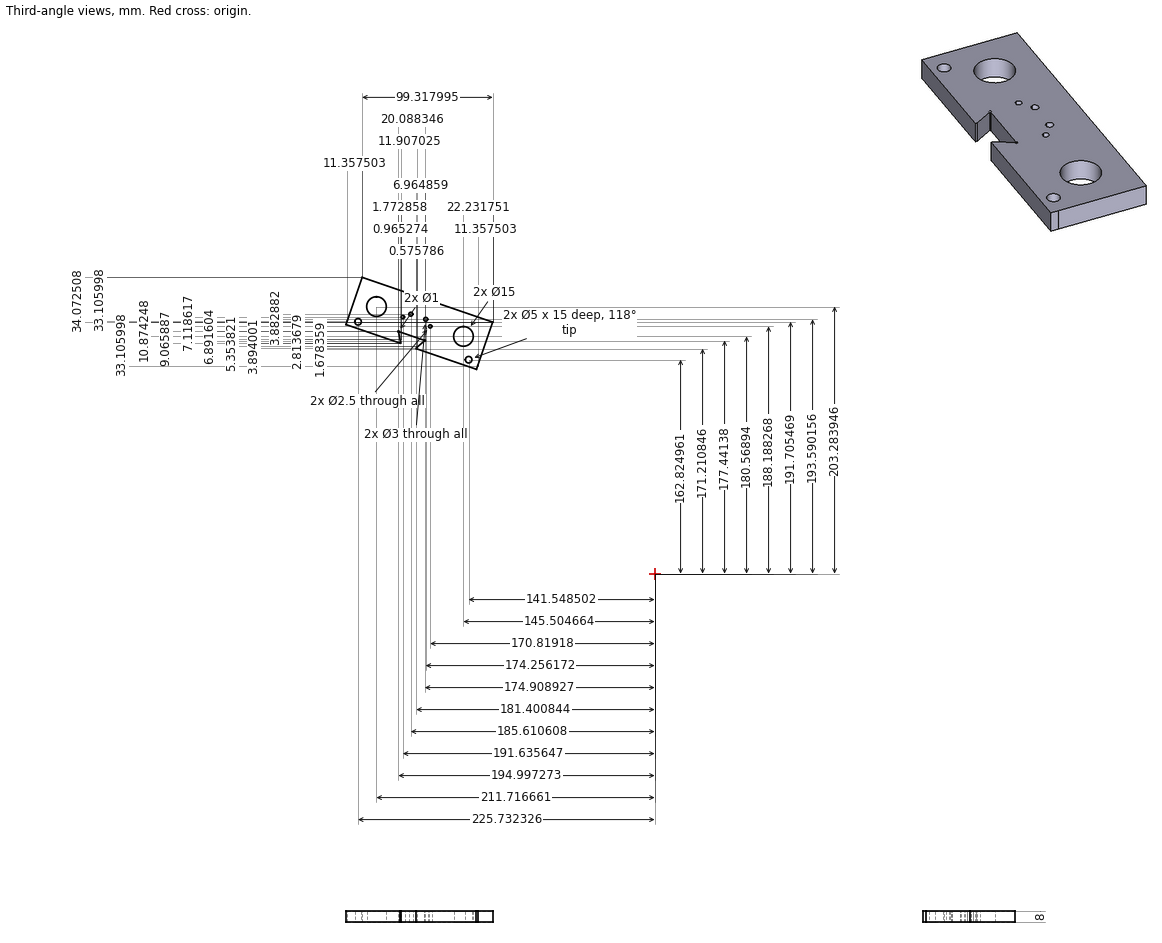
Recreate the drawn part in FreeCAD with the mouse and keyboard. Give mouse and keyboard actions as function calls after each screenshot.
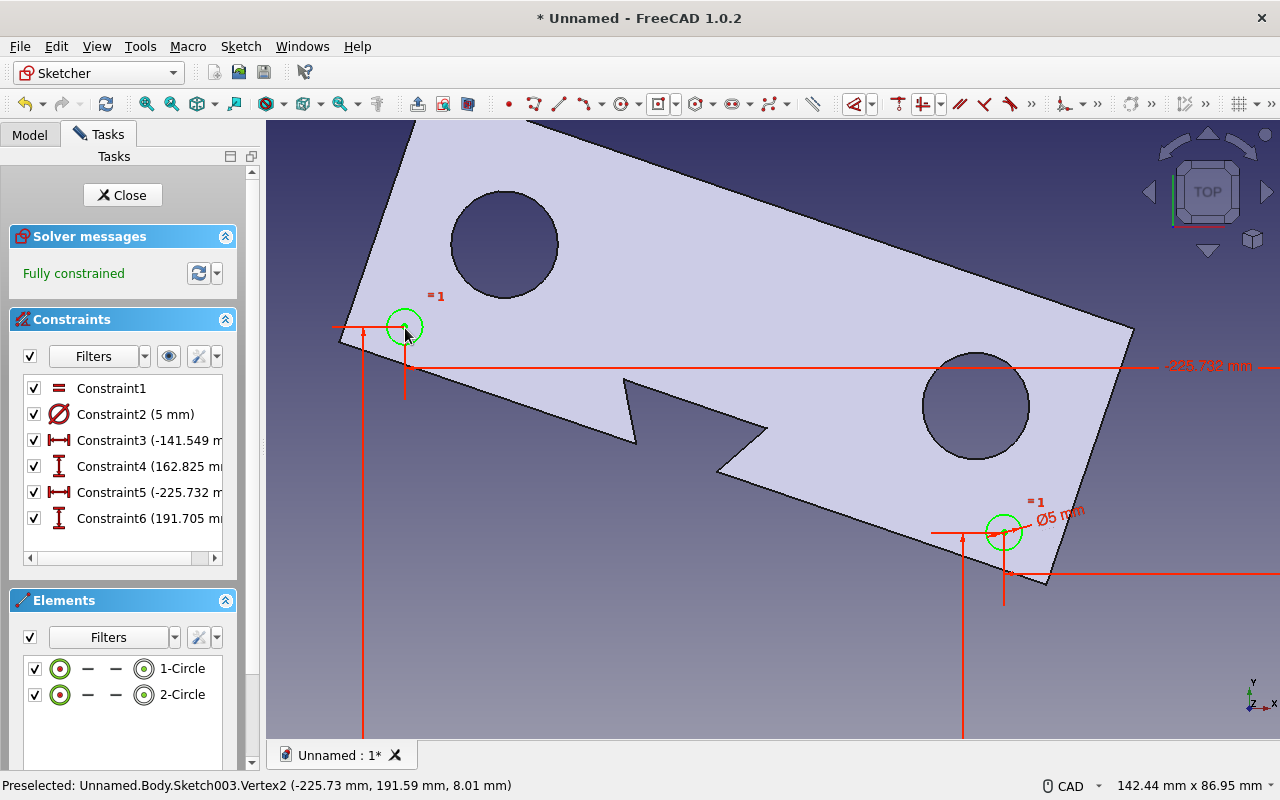
click(123, 195)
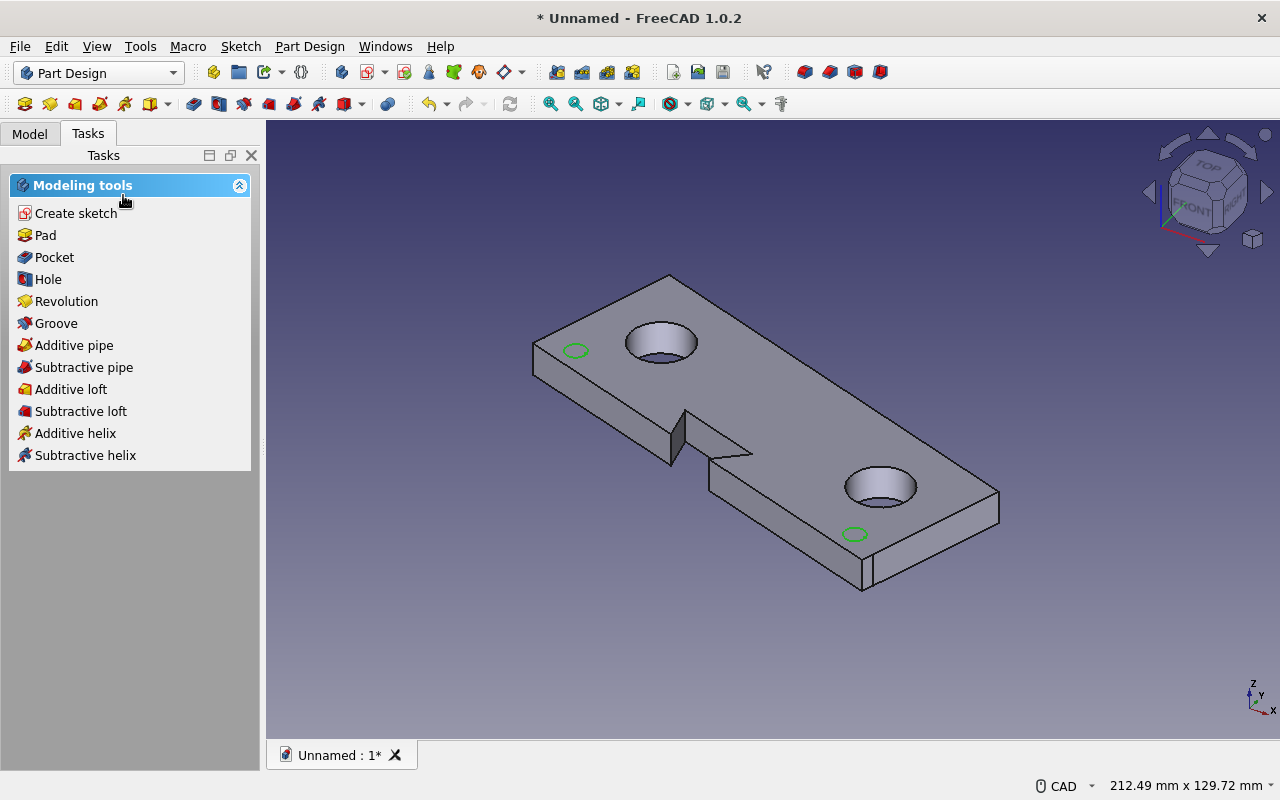
click(219, 104)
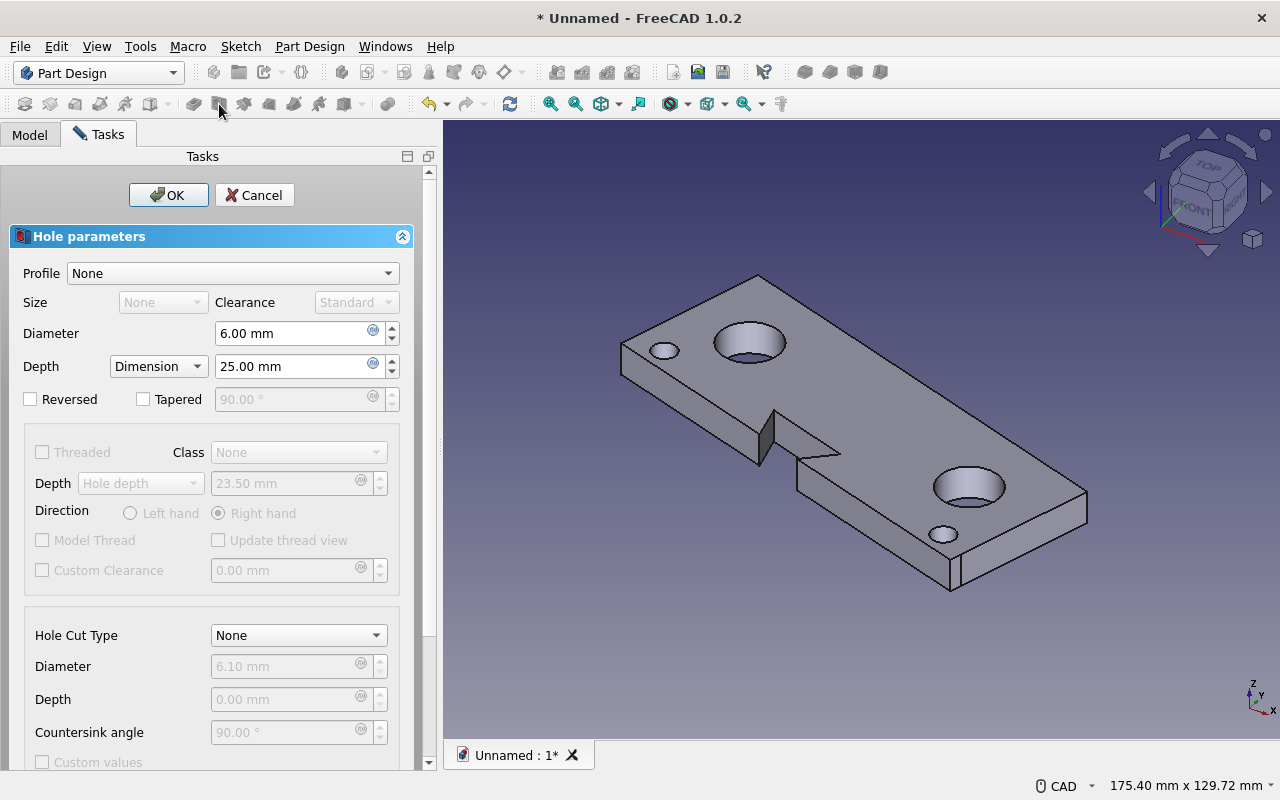
triple_click(300, 334)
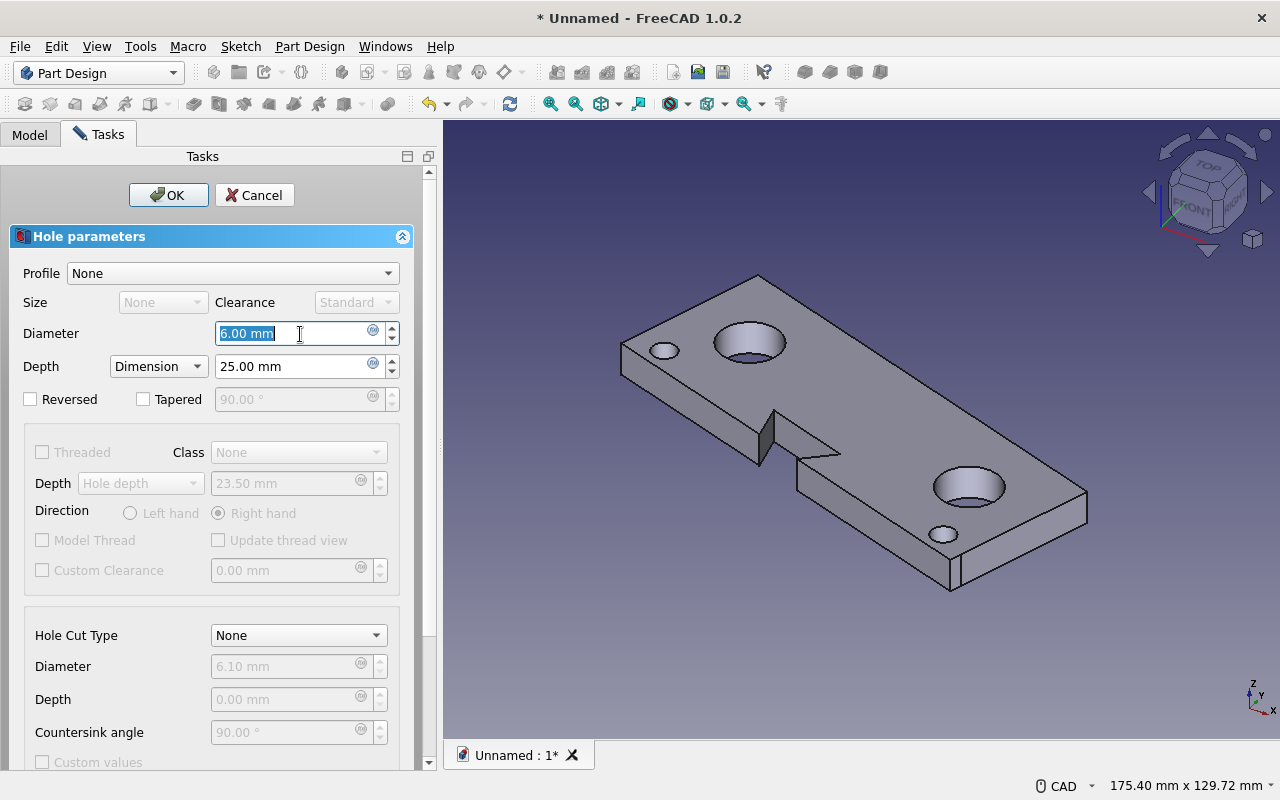
text(5)
key(Tab)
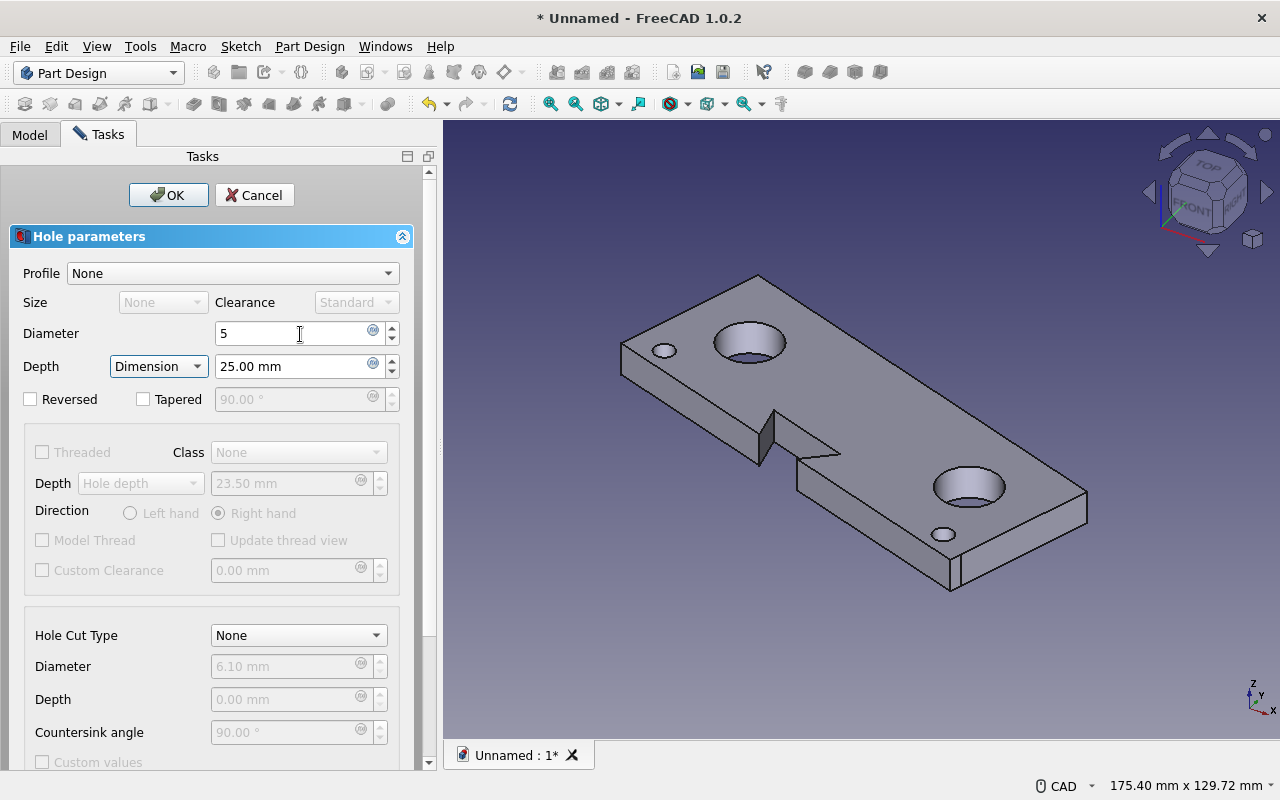
triple_click(300, 366)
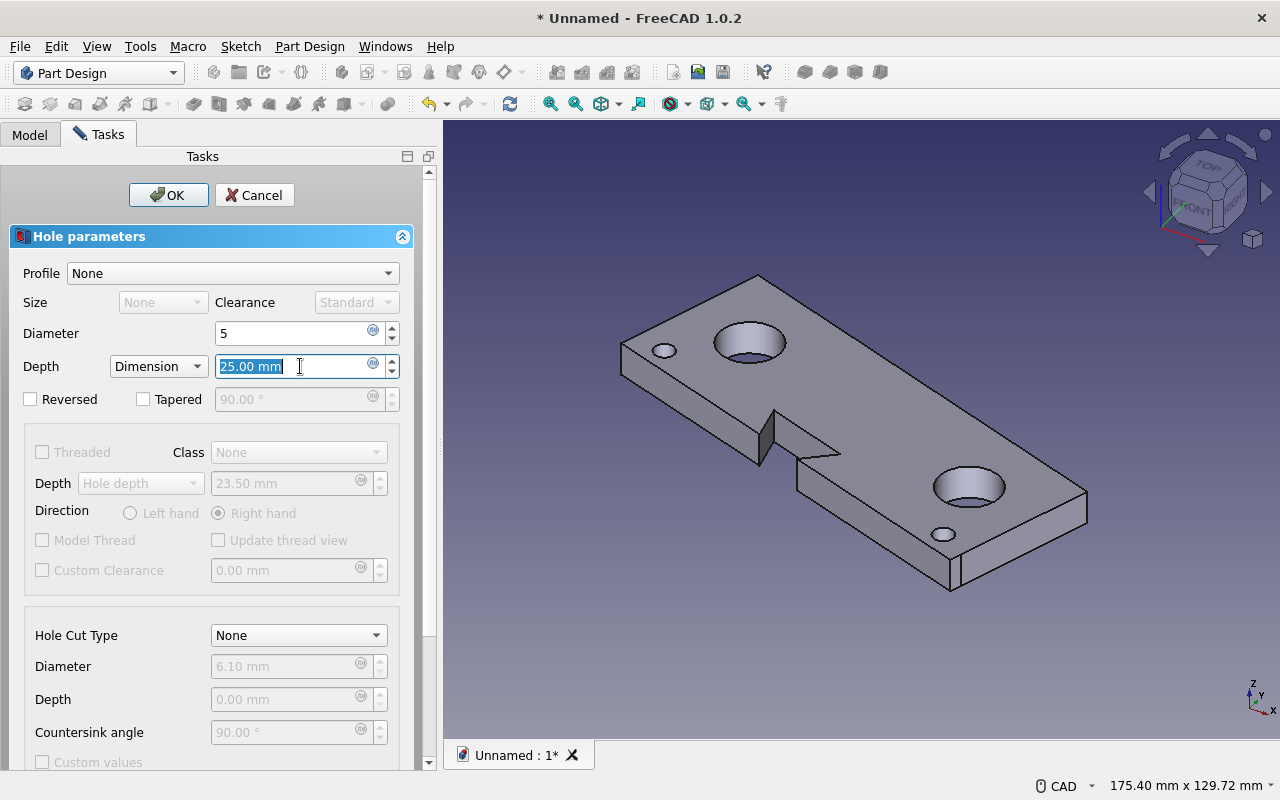
text(15)
key(Tab)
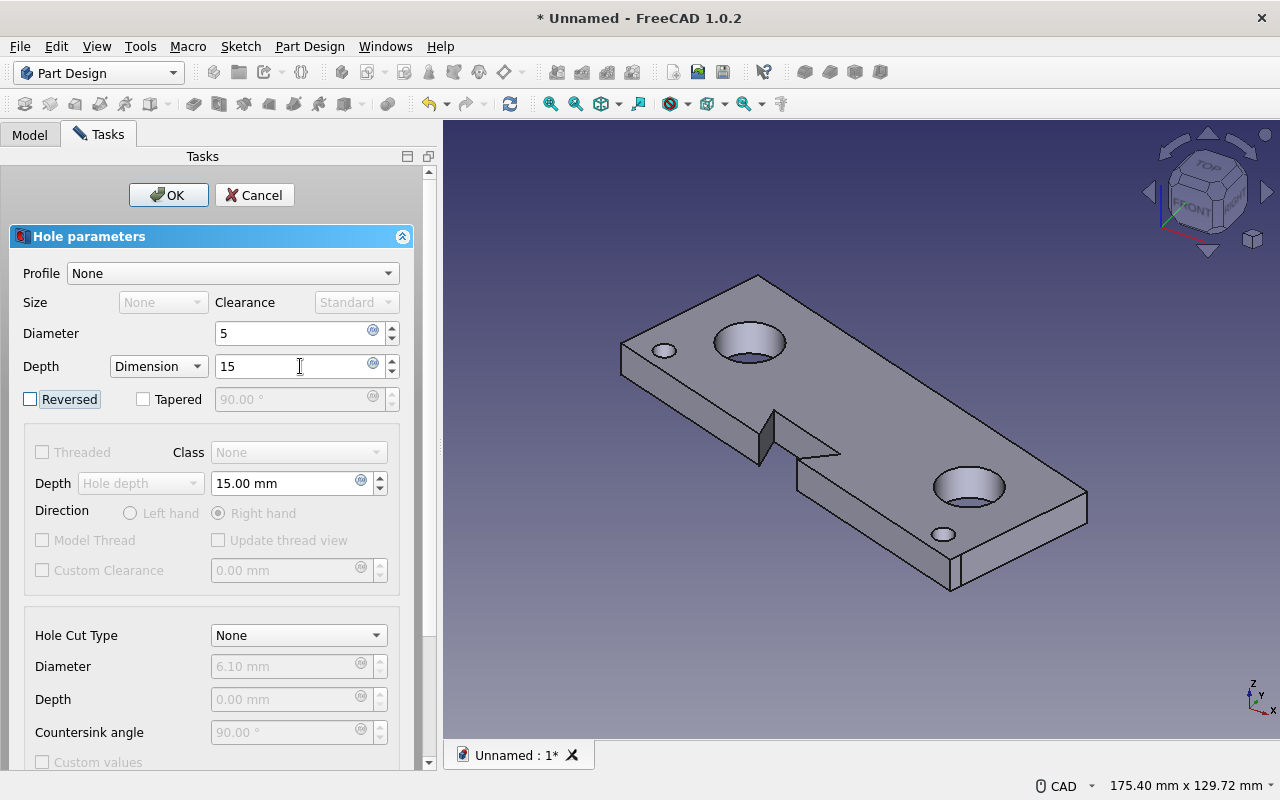
click(169, 195)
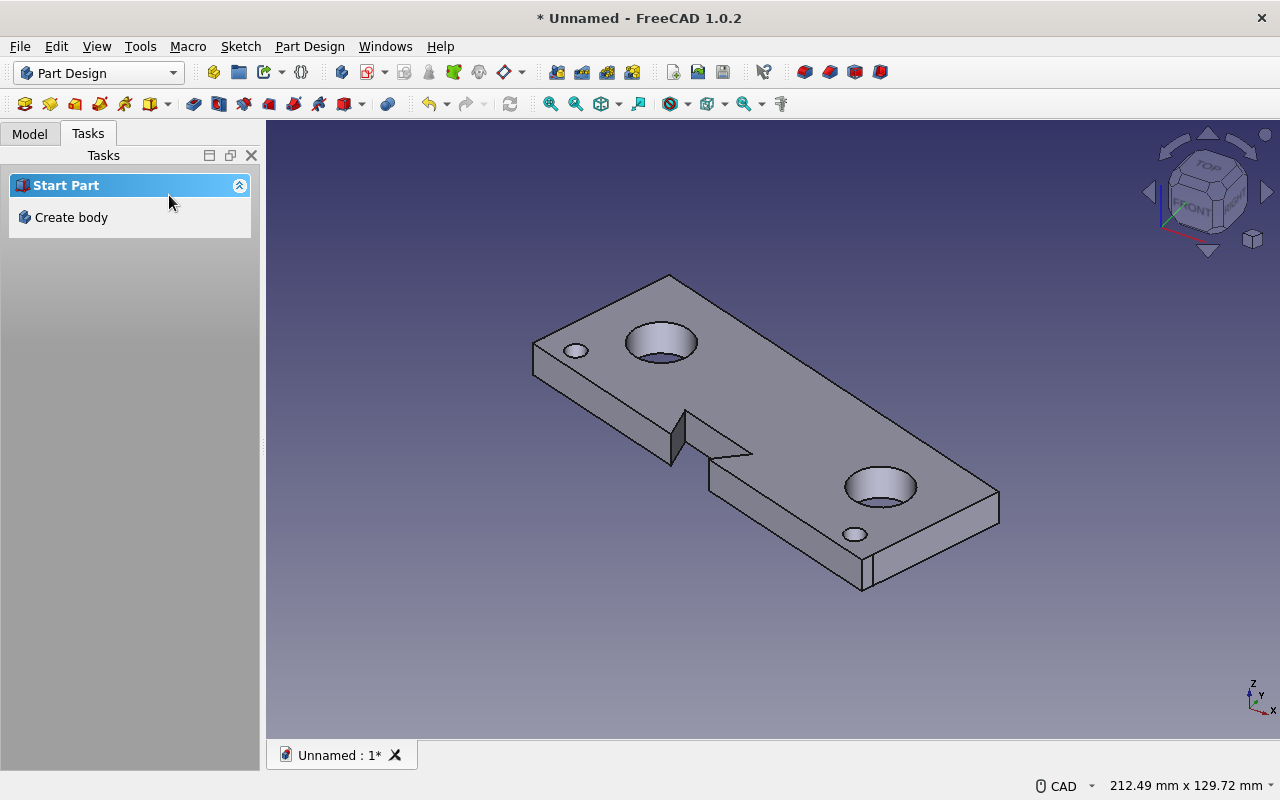
key(5)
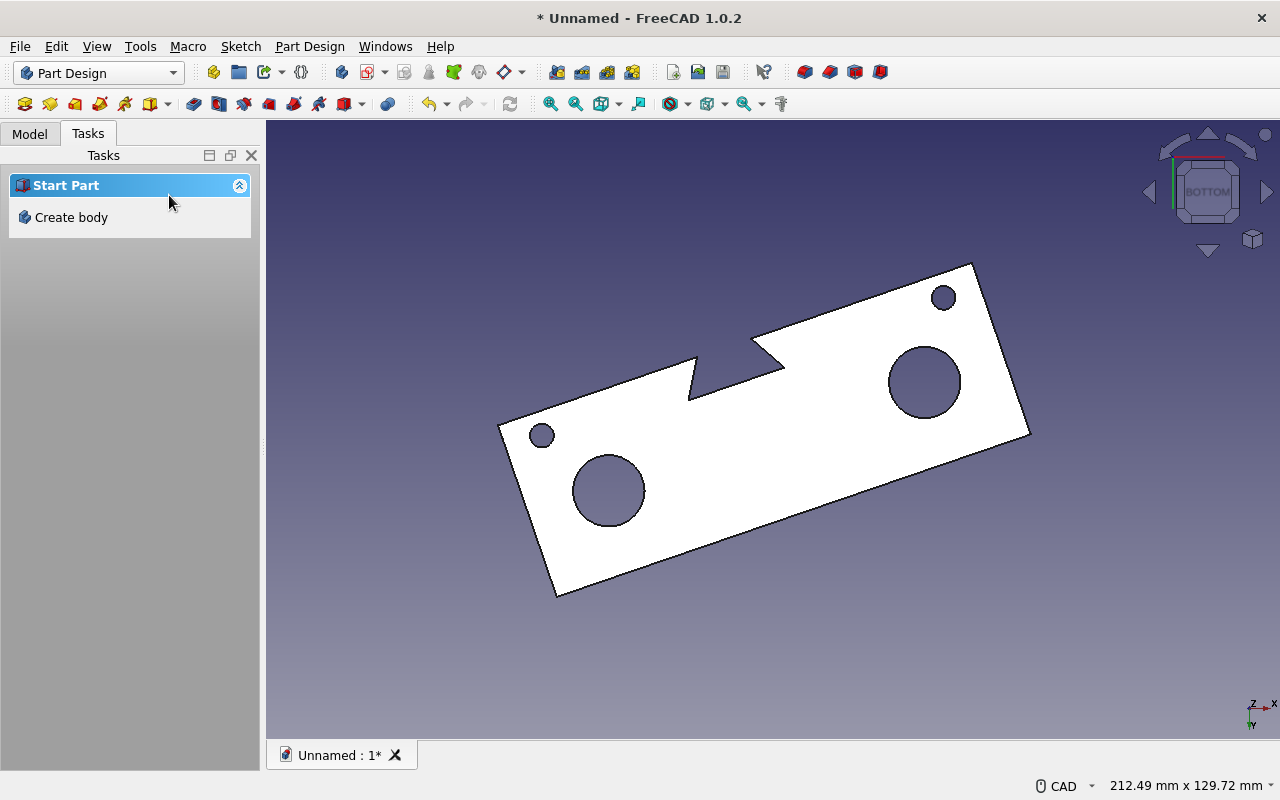
click(840, 429)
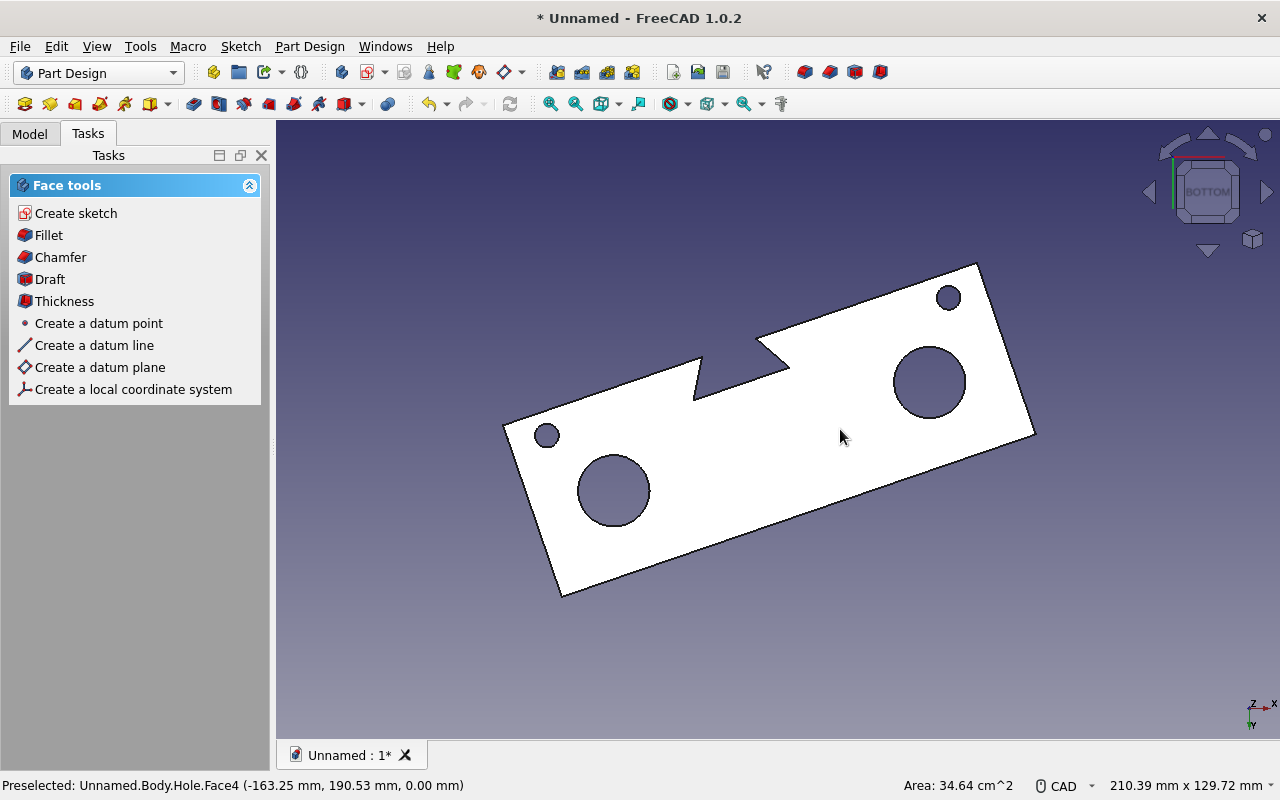
click(366, 72)